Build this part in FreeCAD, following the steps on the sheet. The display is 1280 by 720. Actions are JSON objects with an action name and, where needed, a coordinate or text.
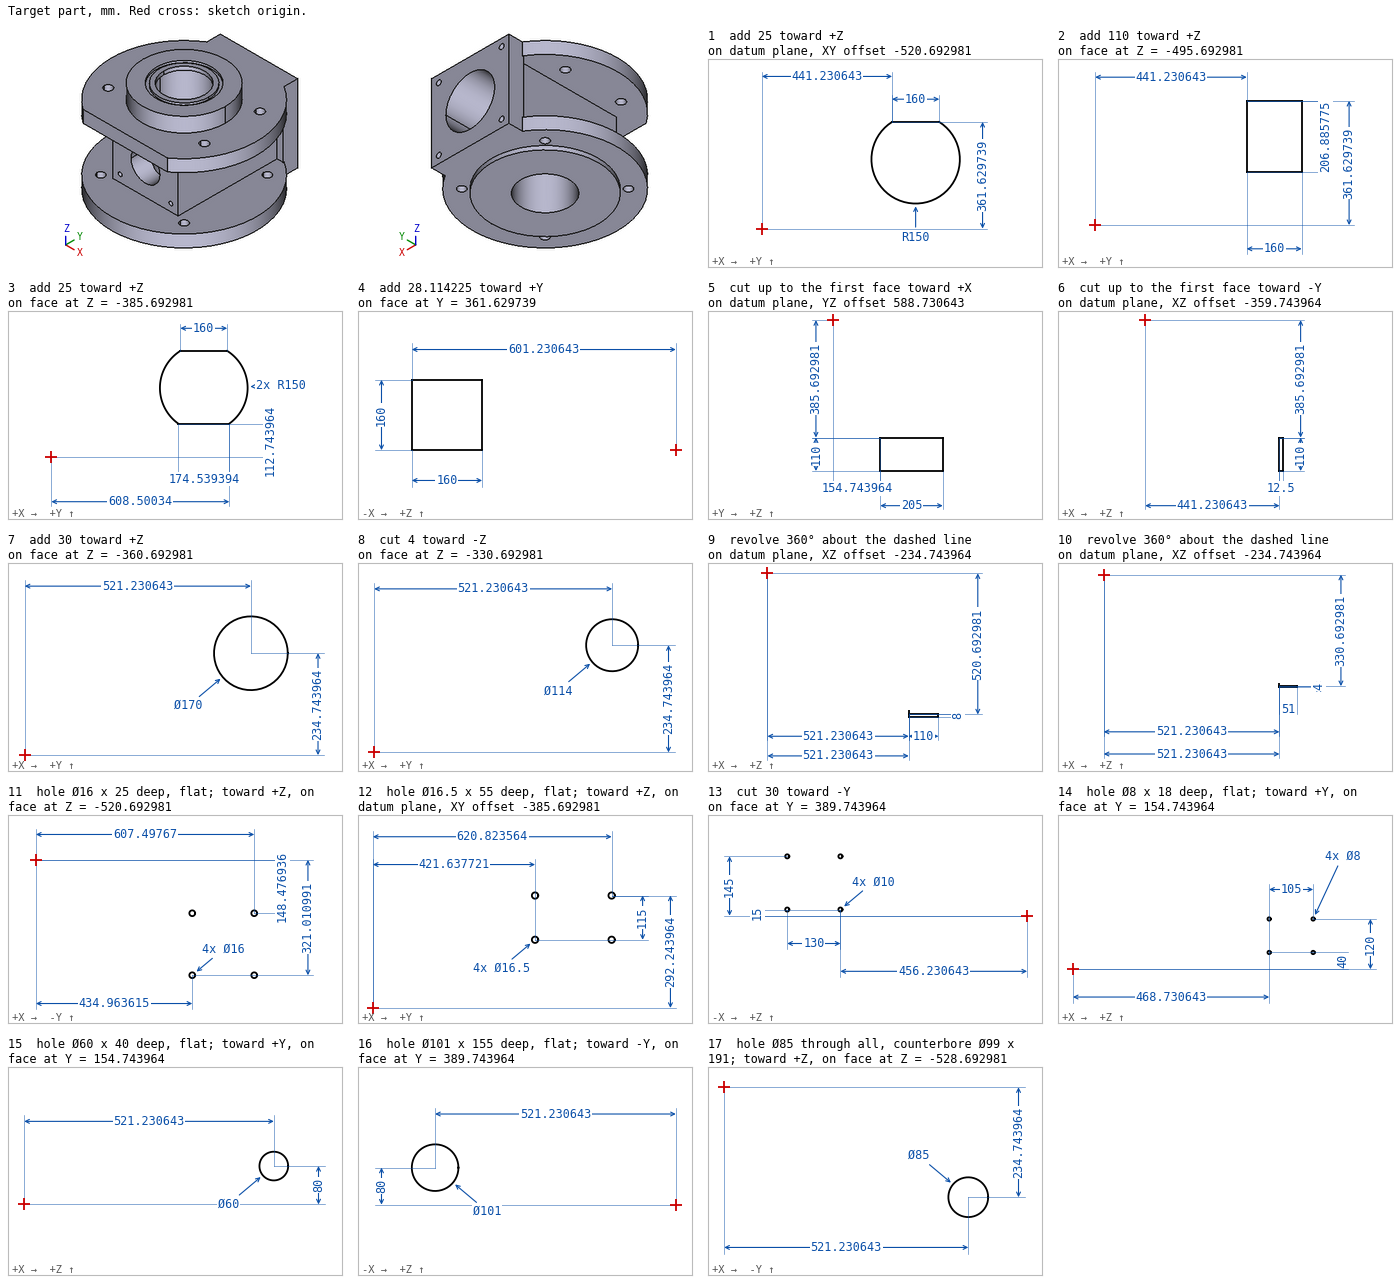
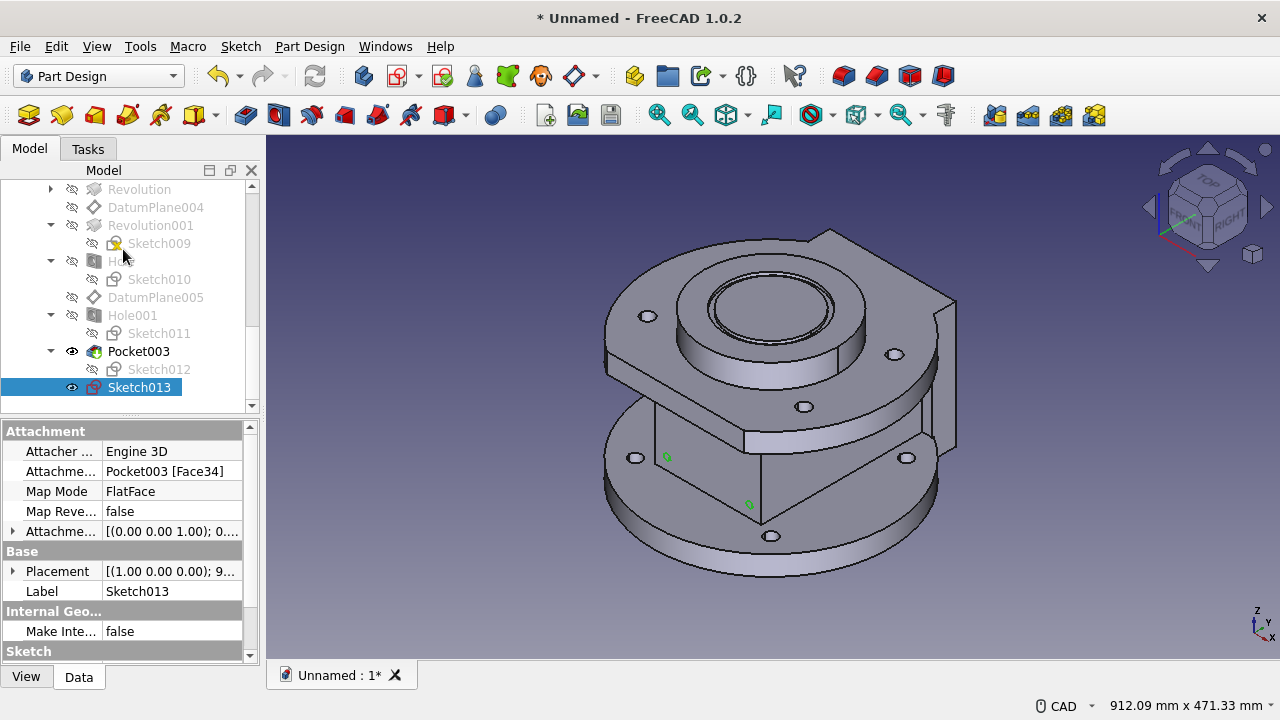
{"action": "left_click", "coordinate": [279, 116]}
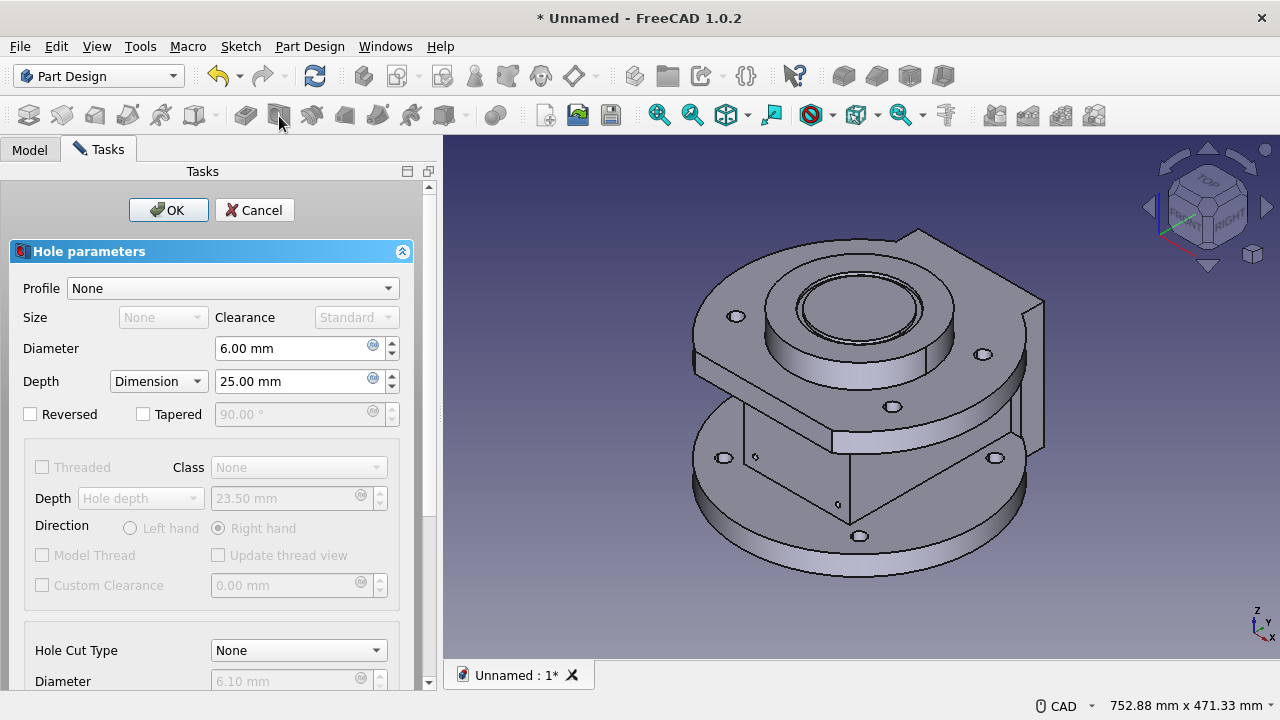
{"action": "triple_click", "coordinate": [300, 348]}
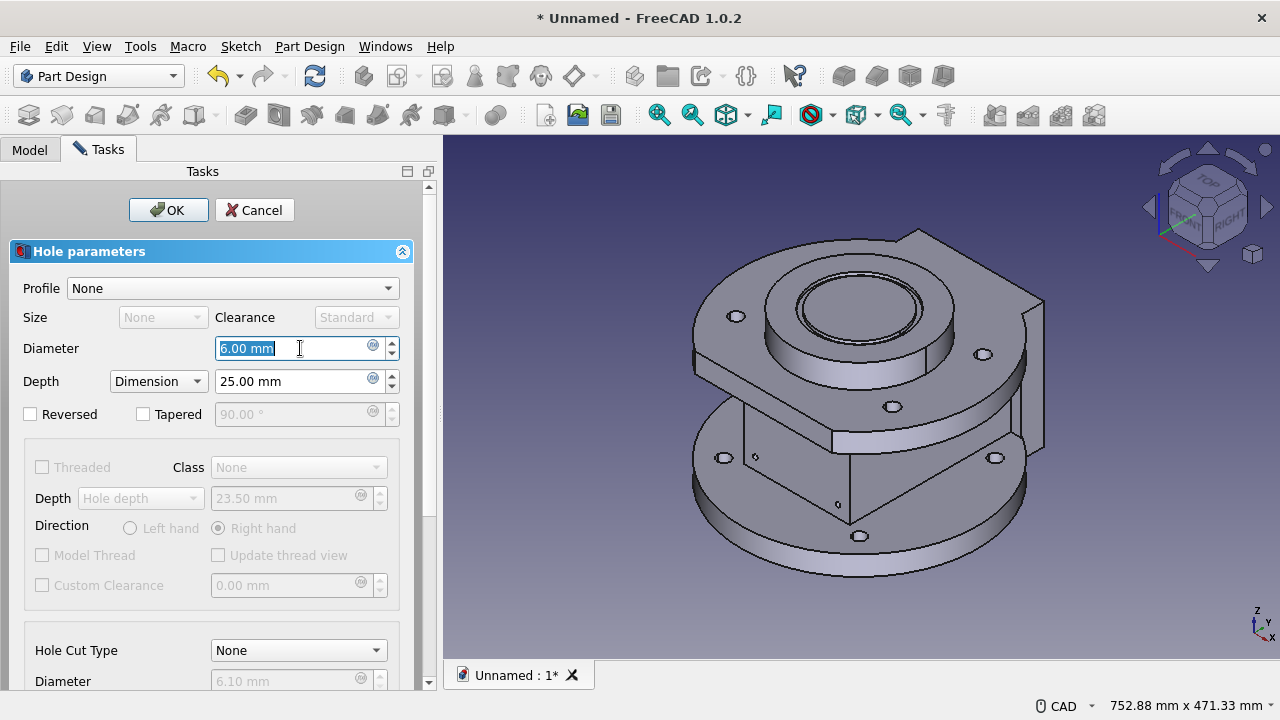
{"action": "type", "text": "8"}
{"action": "key", "text": "Tab"}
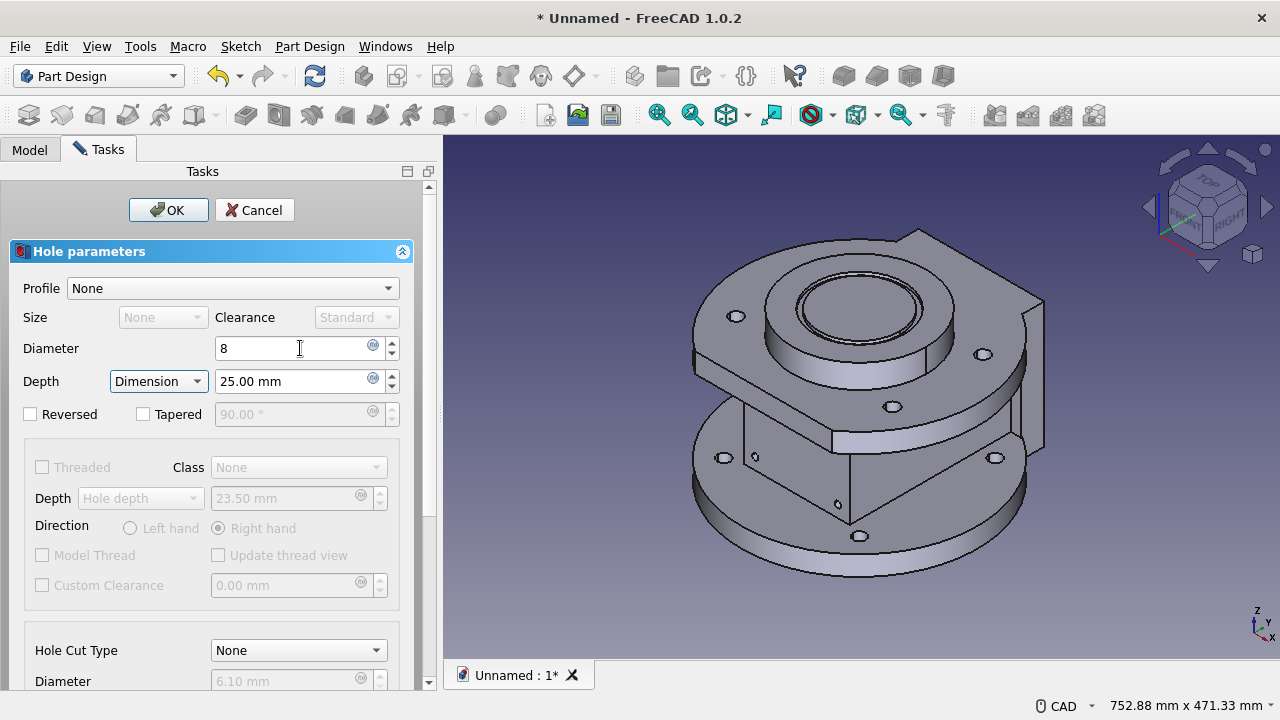
{"action": "triple_click", "coordinate": [300, 382]}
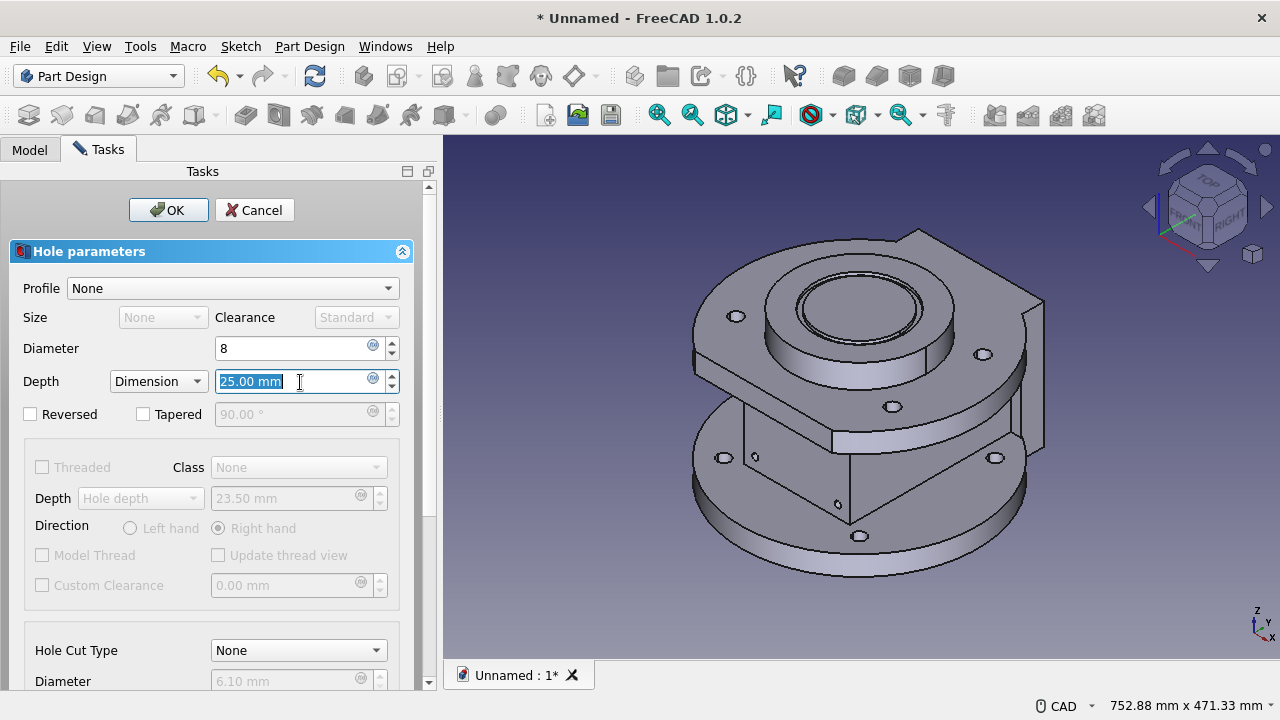
{"action": "type", "text": "18"}
{"action": "key", "text": "Tab"}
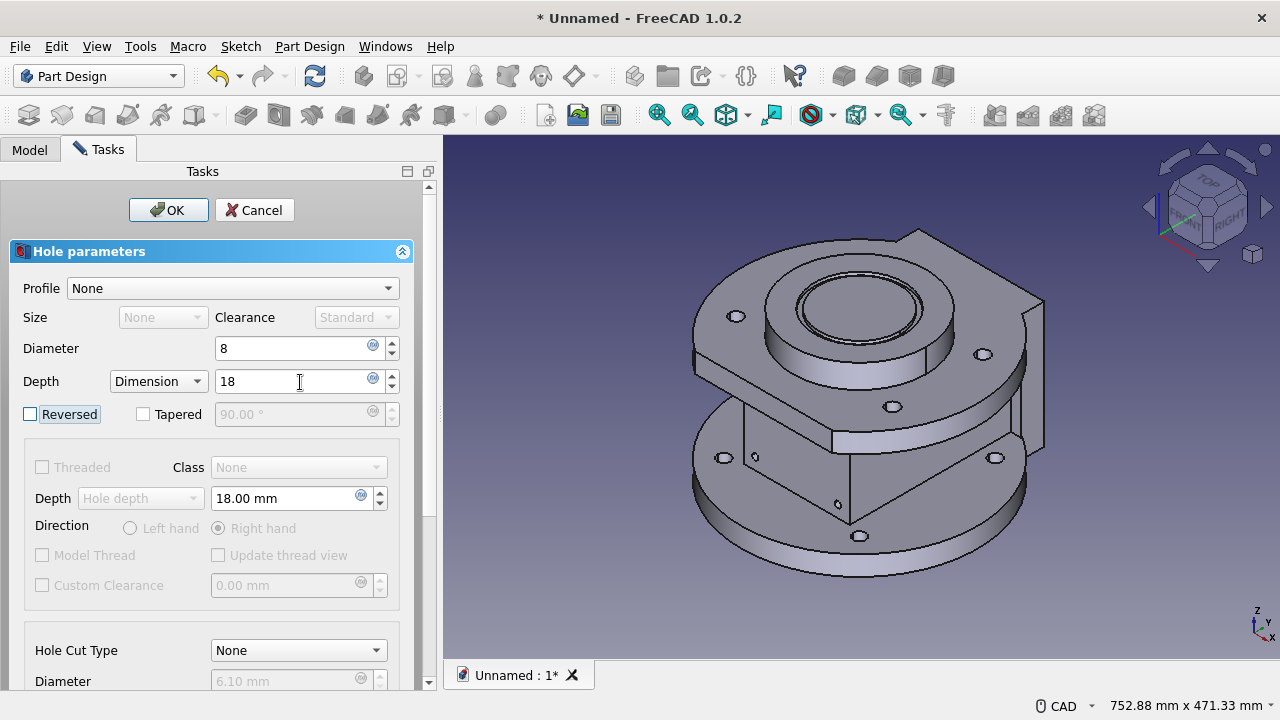
{"action": "scroll", "coordinate": [429, 436], "scroll_direction": "down", "scroll_amount": 4}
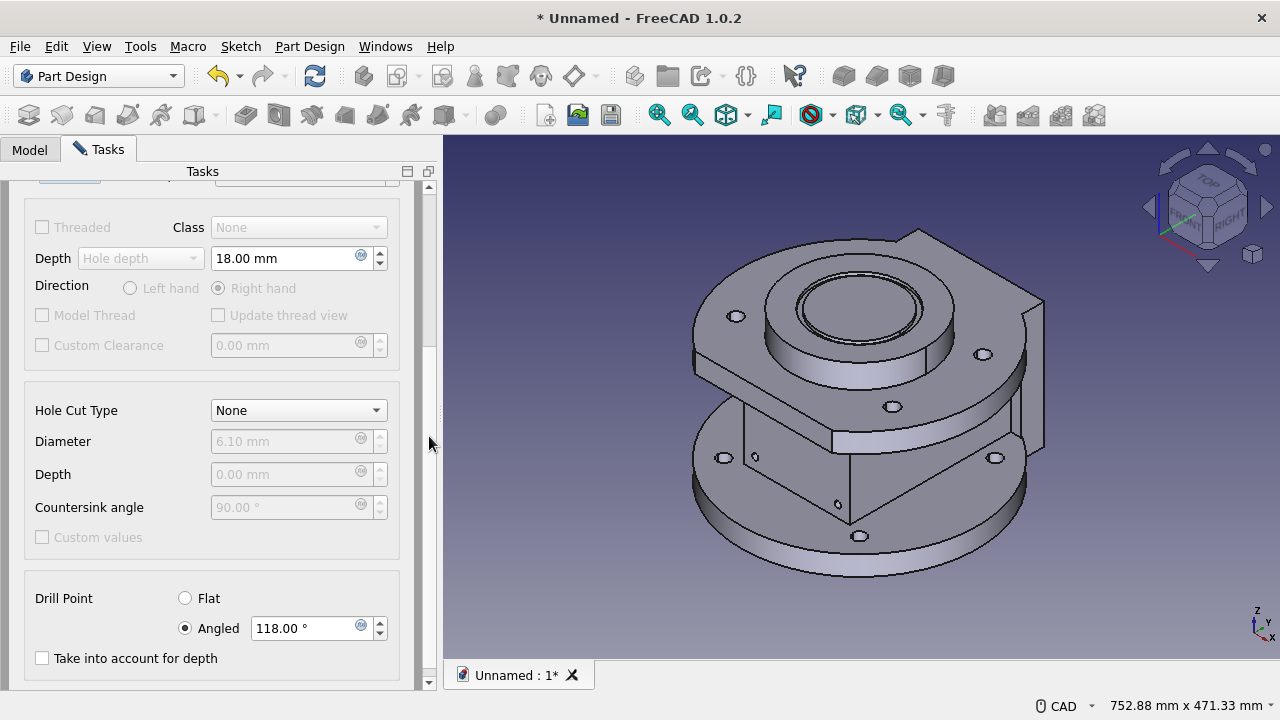
{"action": "left_click", "coordinate": [186, 596]}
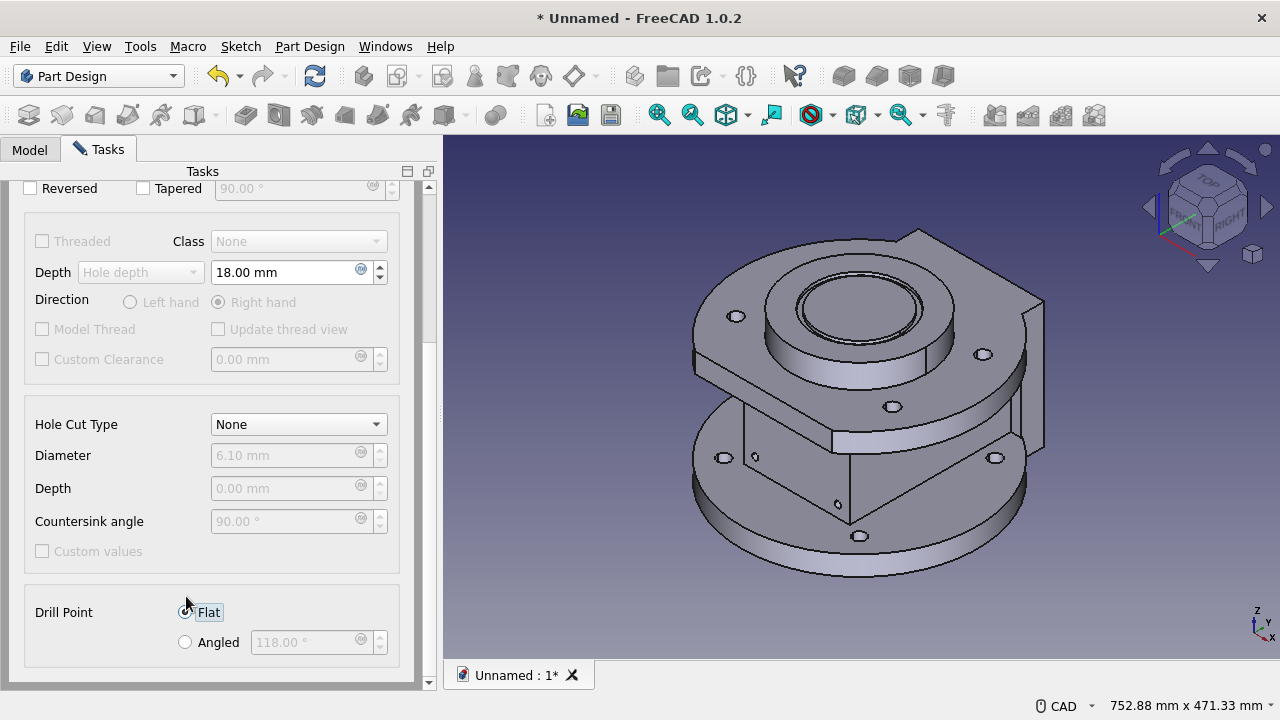
{"action": "scroll", "coordinate": [429, 436], "scroll_direction": "up", "scroll_amount": 5}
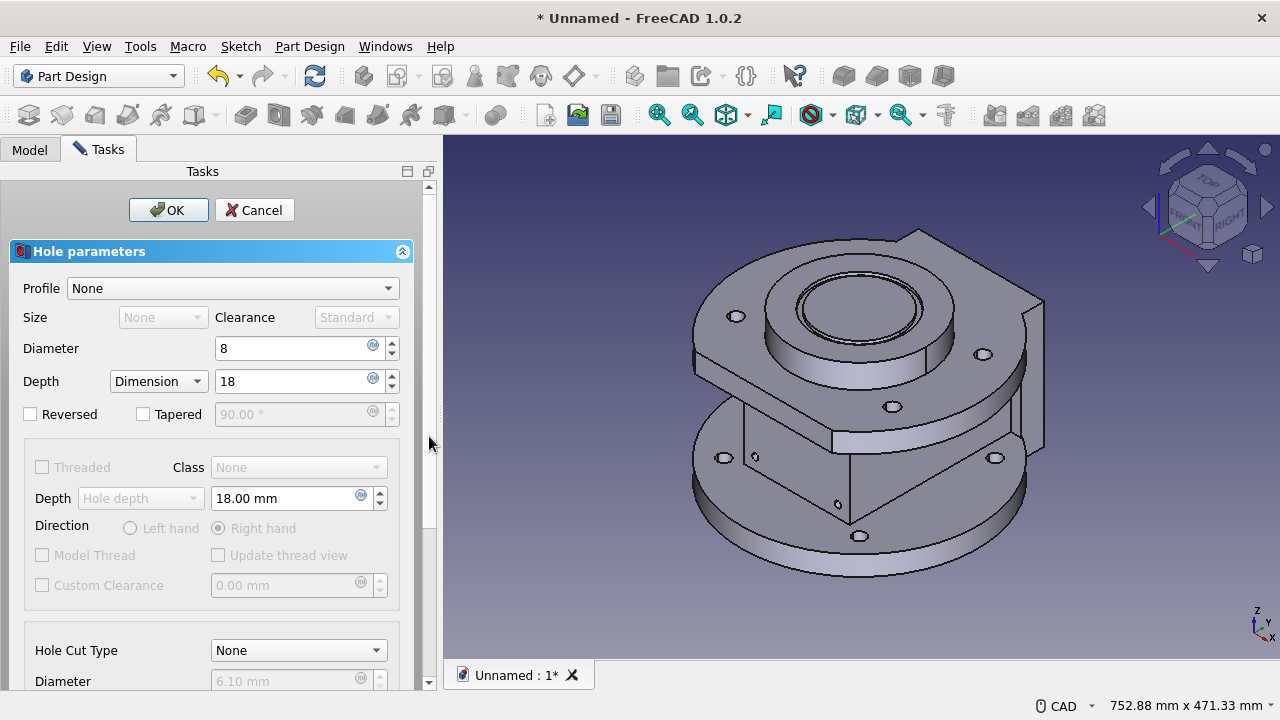
{"action": "left_click", "coordinate": [169, 210]}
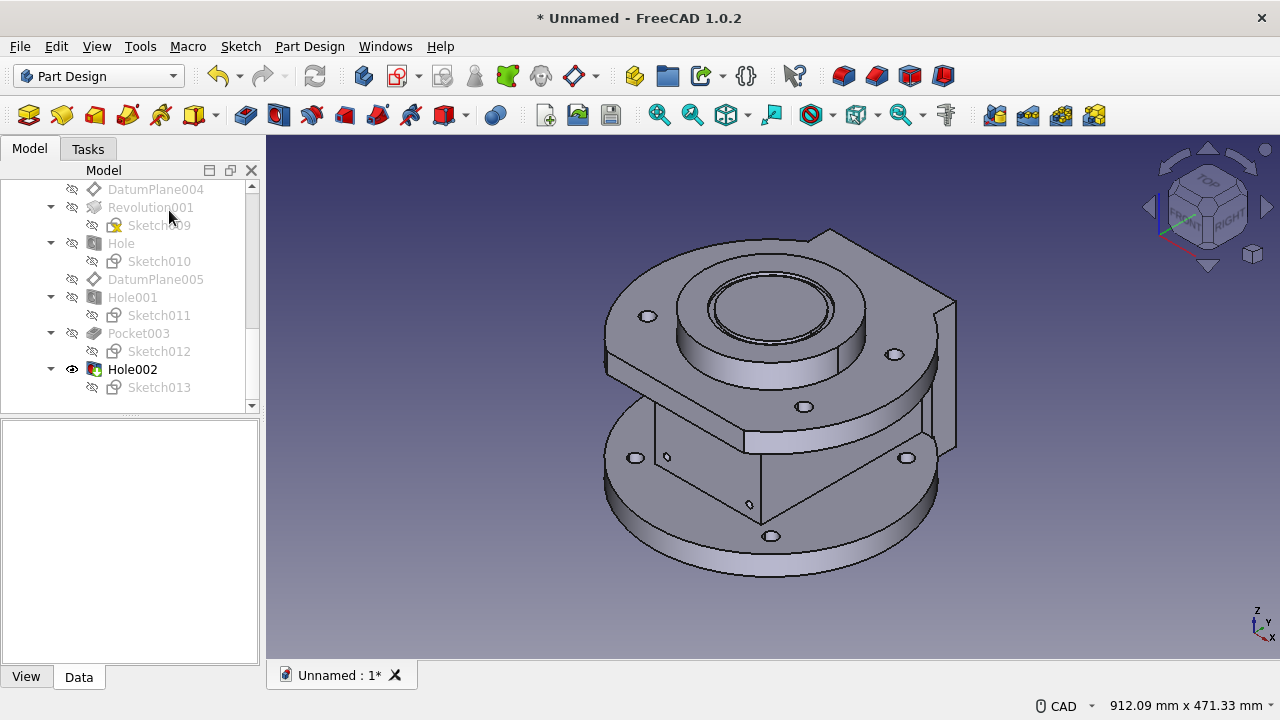
{"action": "left_click", "coordinate": [708, 443]}